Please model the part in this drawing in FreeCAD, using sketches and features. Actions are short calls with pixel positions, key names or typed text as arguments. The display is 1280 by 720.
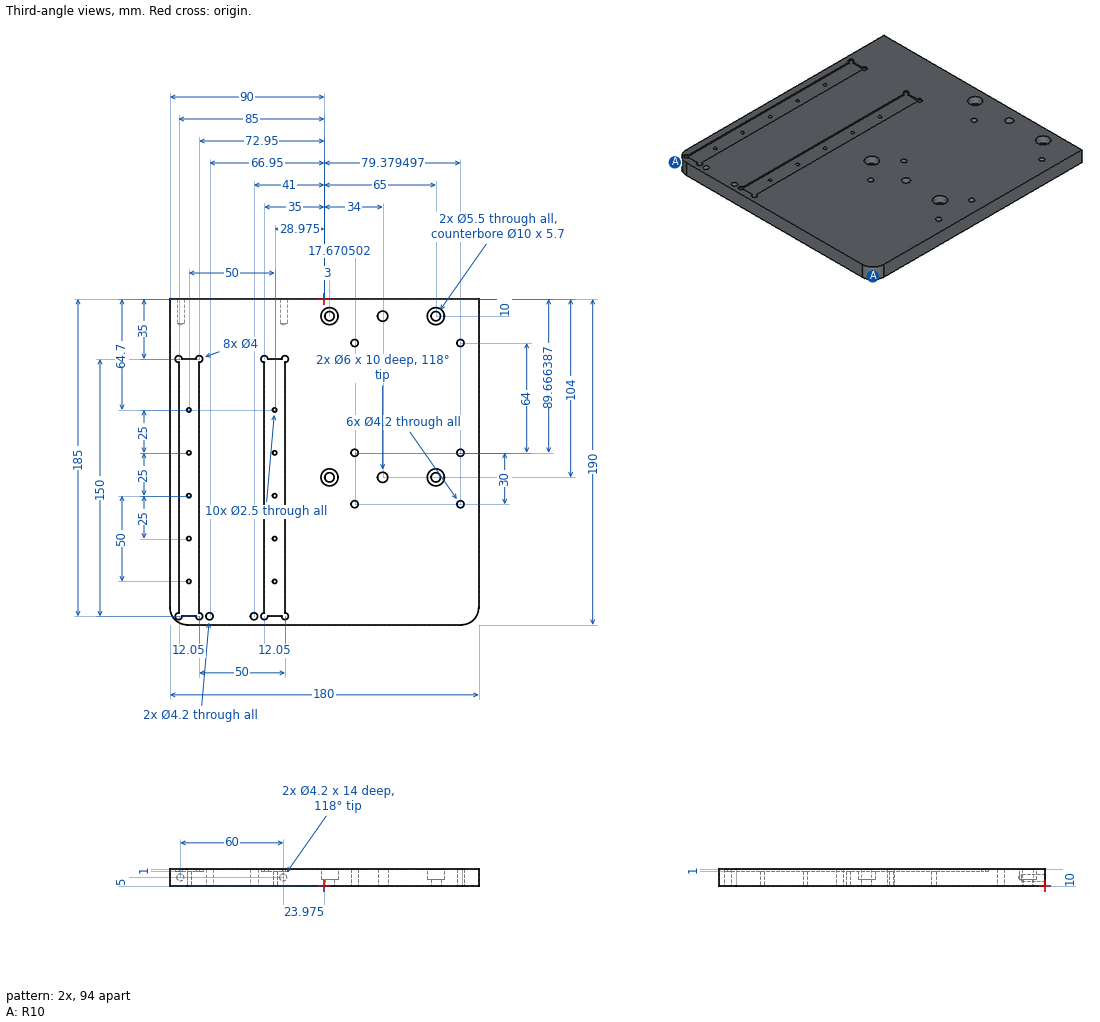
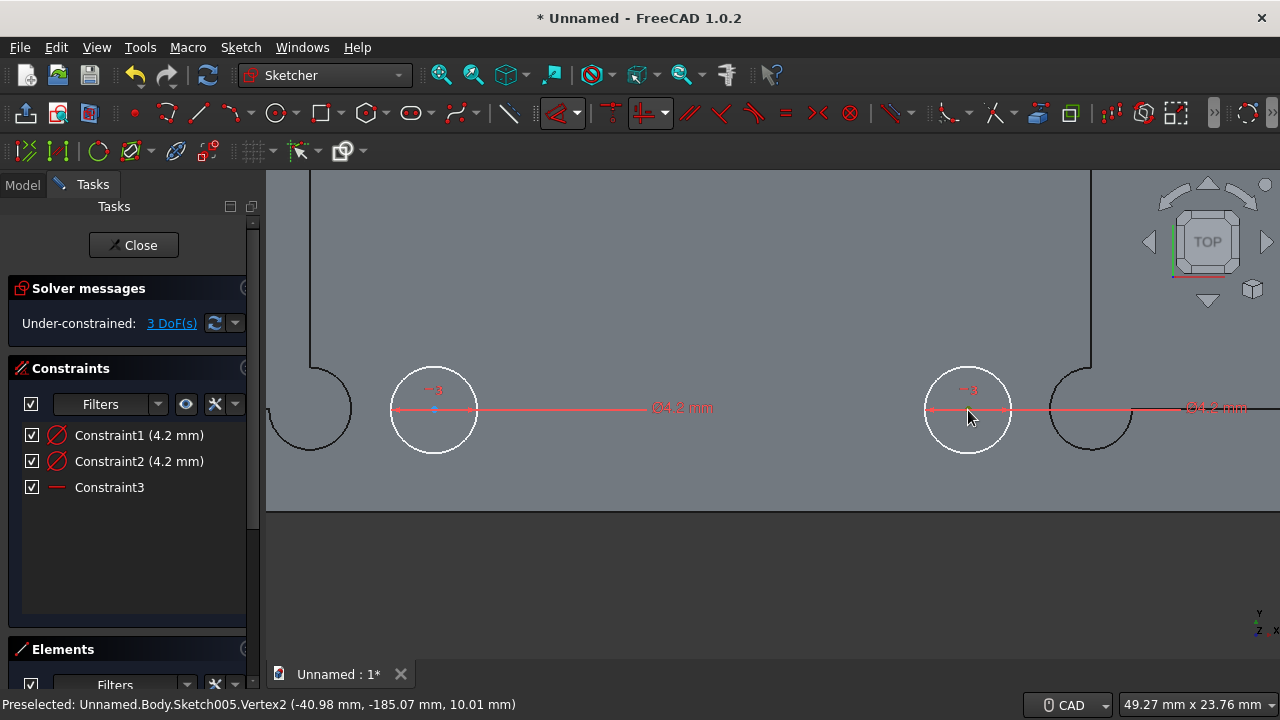
click(580, 114)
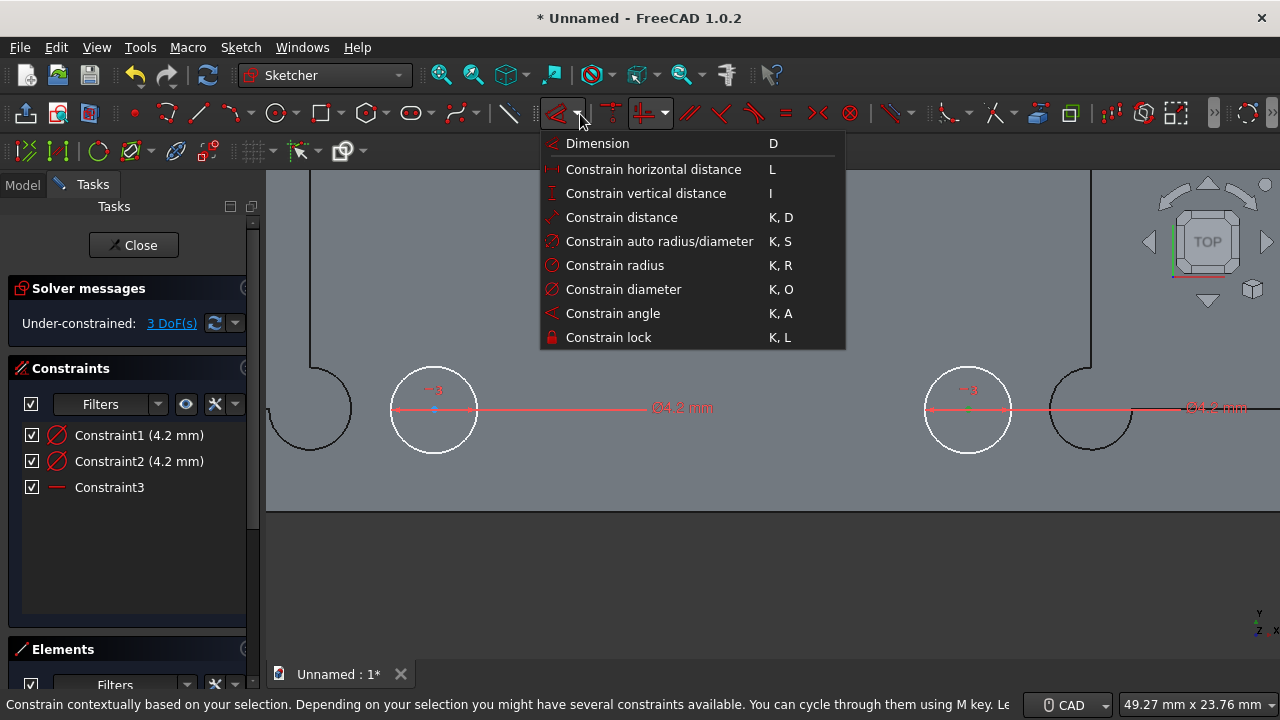
click(693, 169)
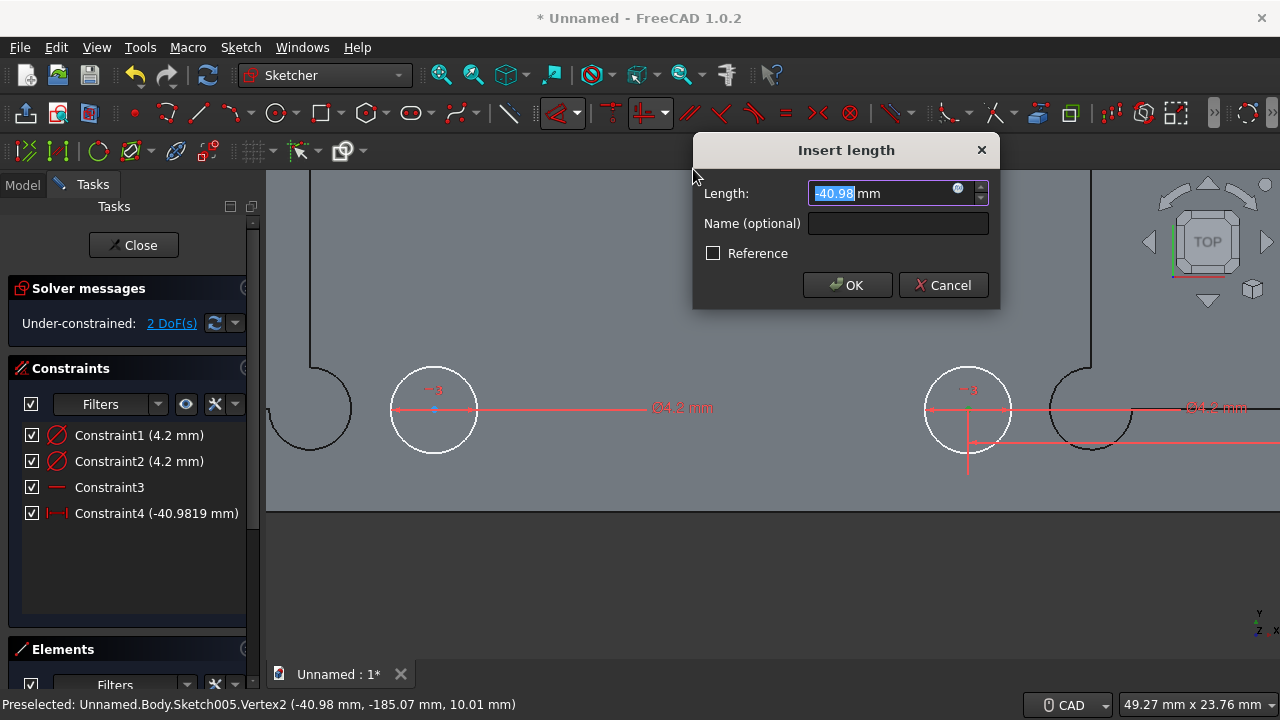
text(-41)
key(Return)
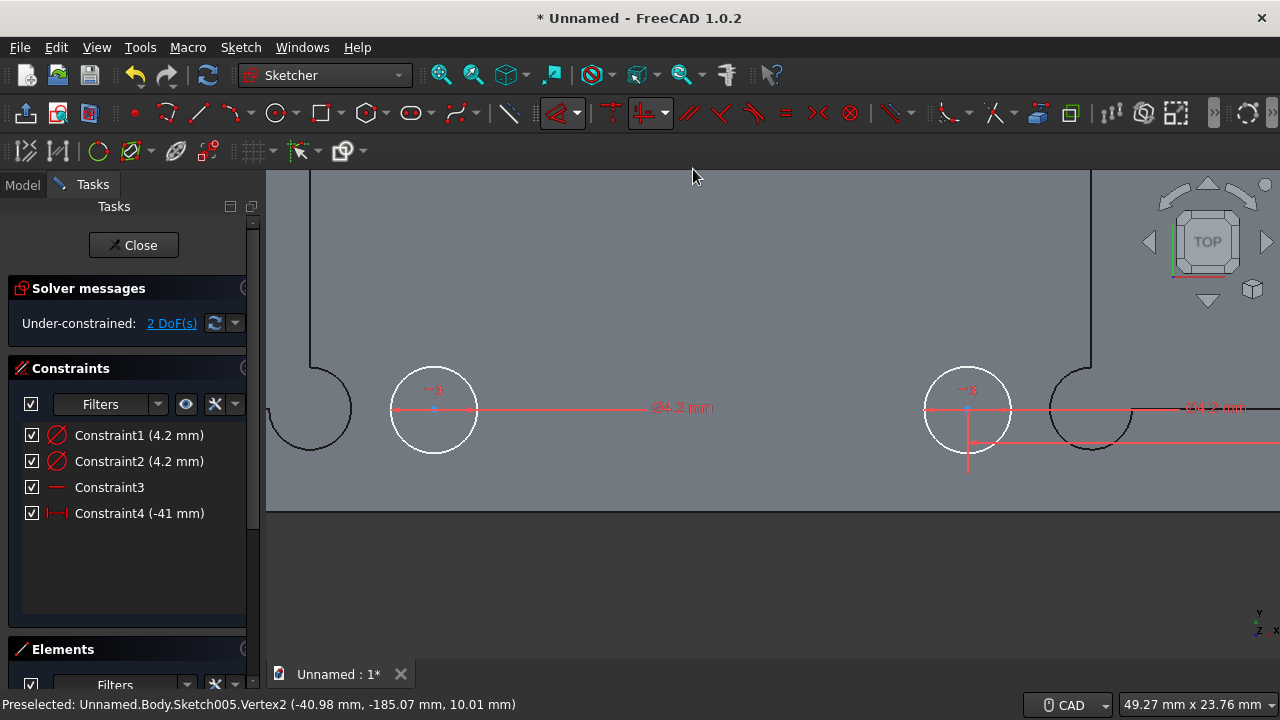
click(434, 410)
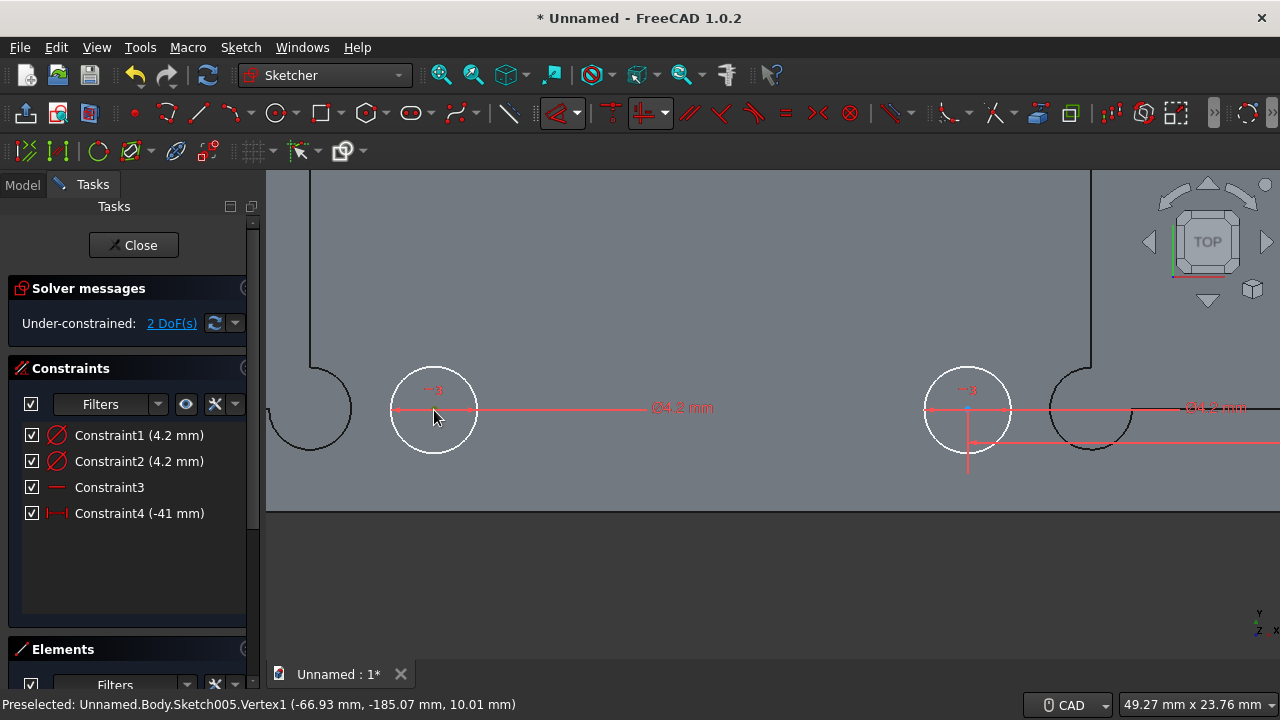
key(i)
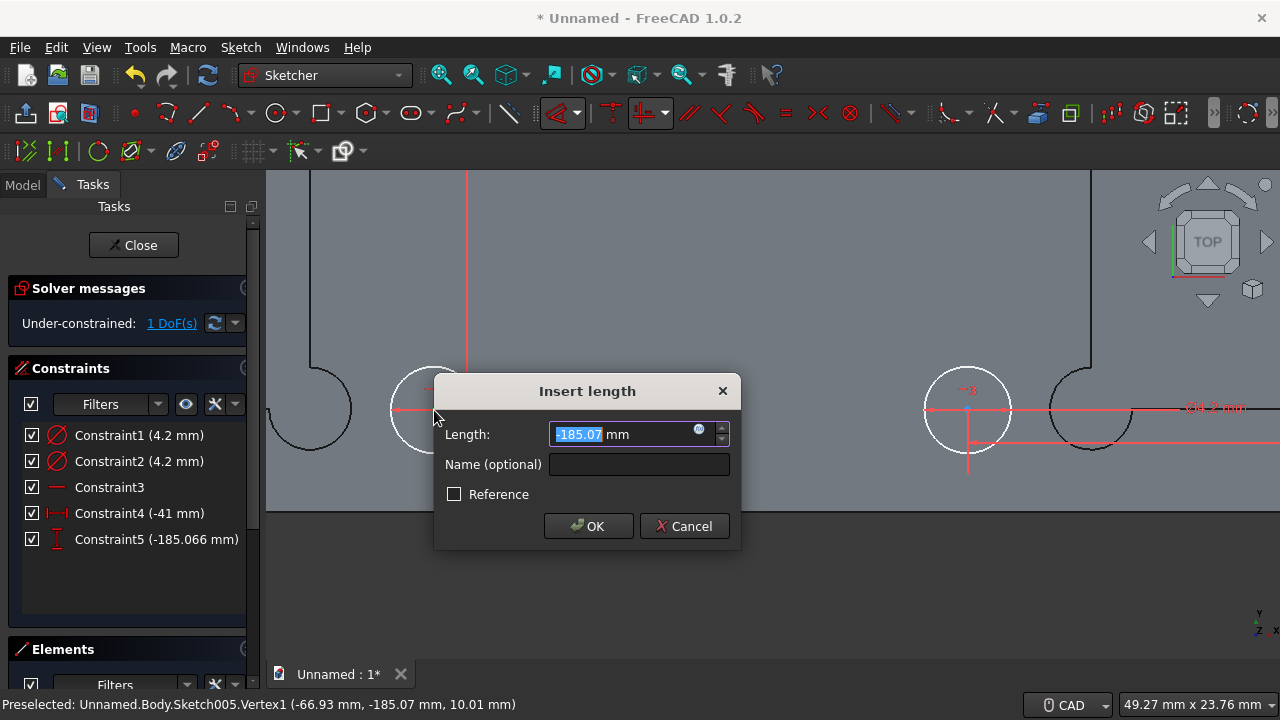
text(-185)
key(Return)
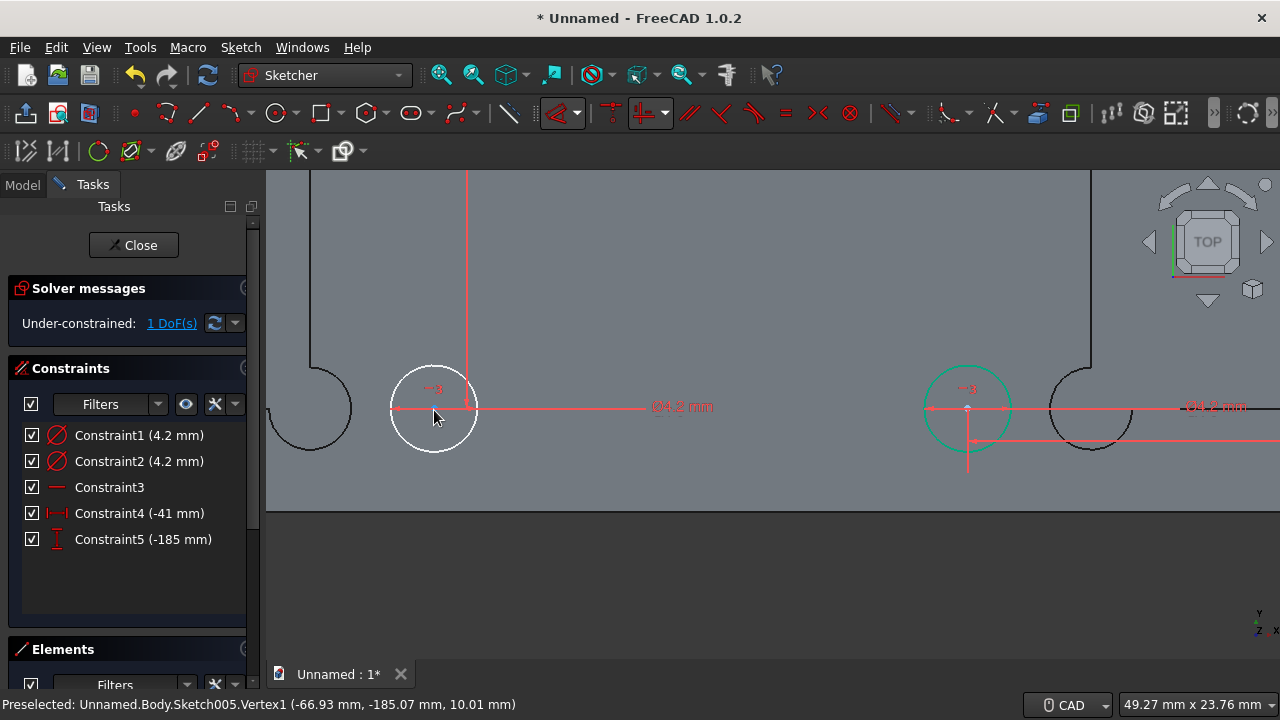
click(434, 409)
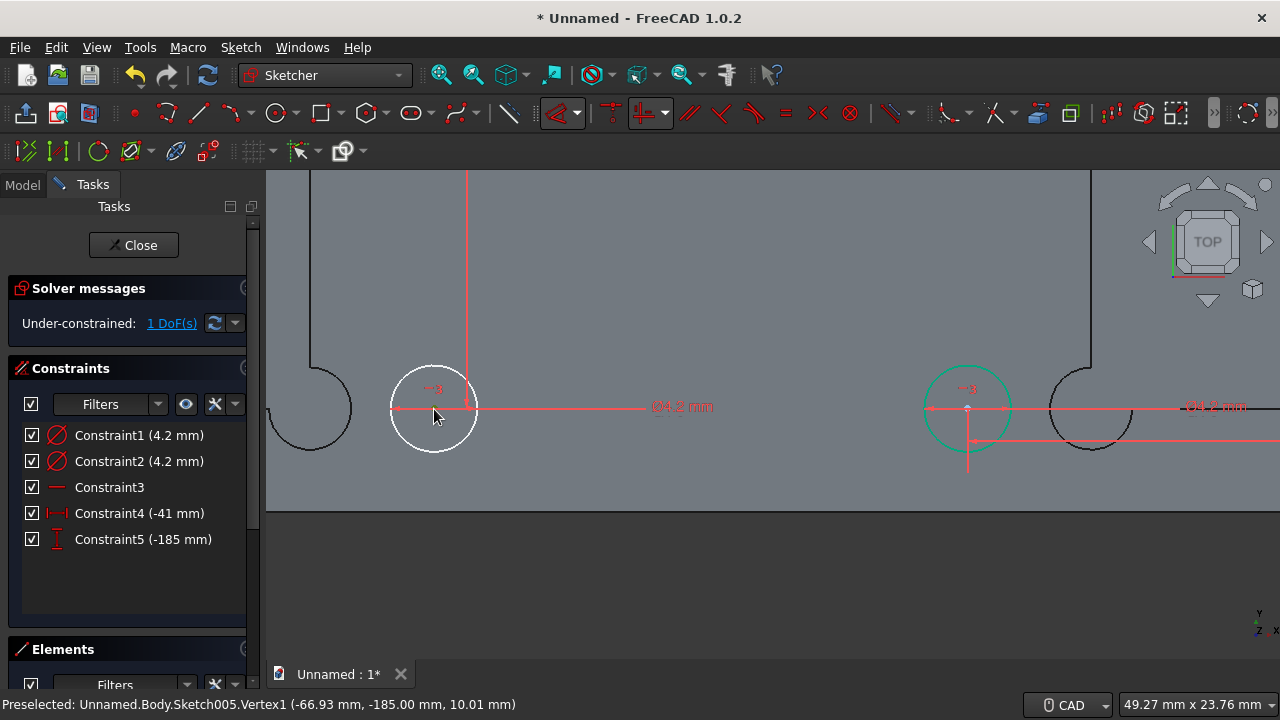
key(l)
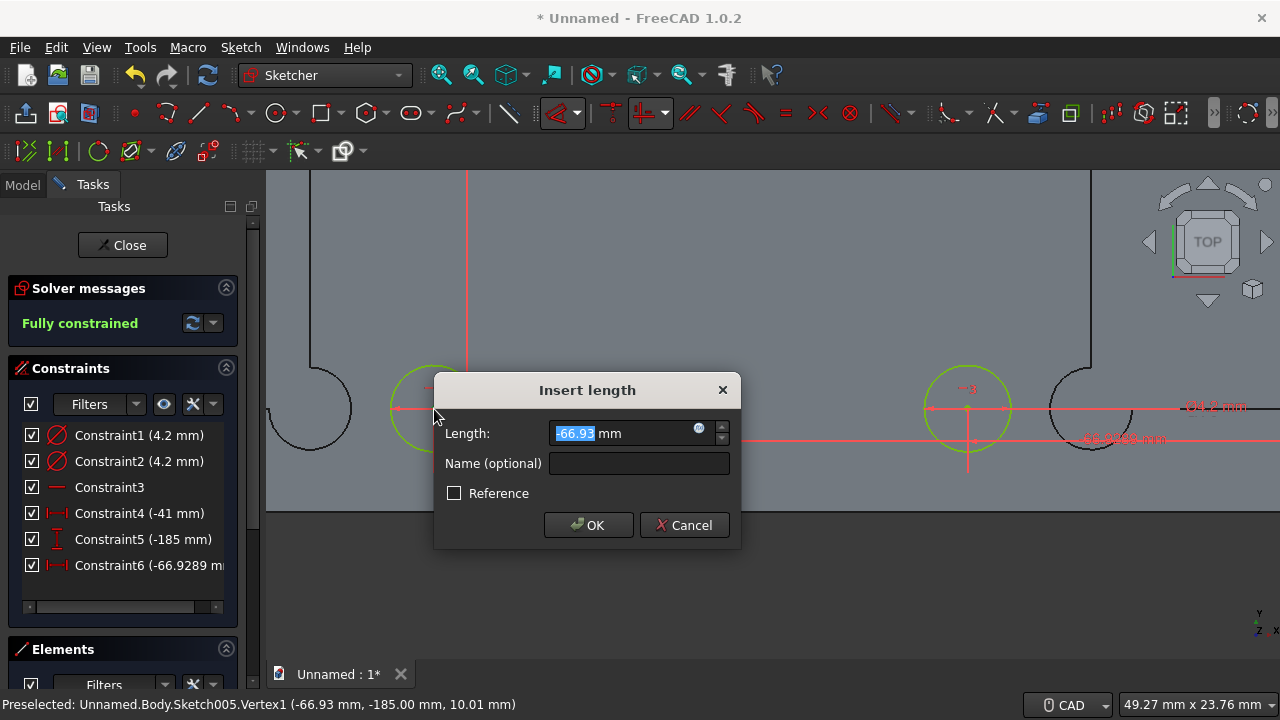
text(-66.95)
key(Return)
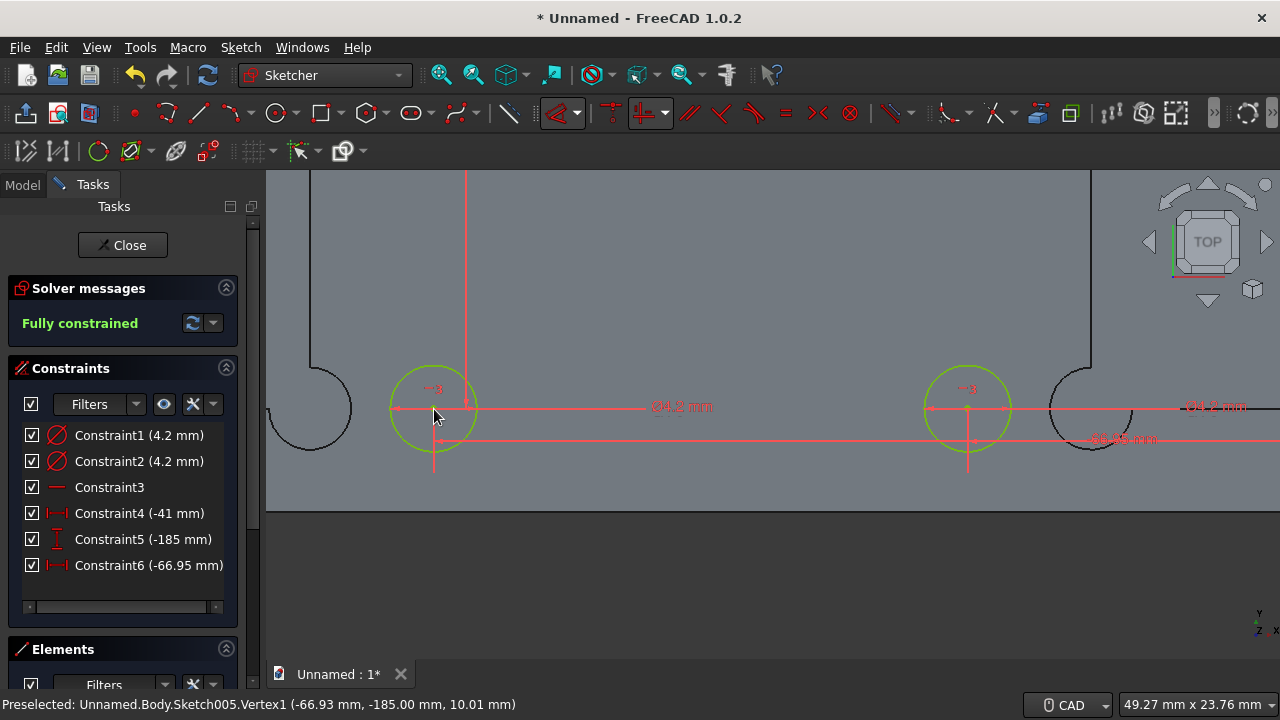
click(123, 245)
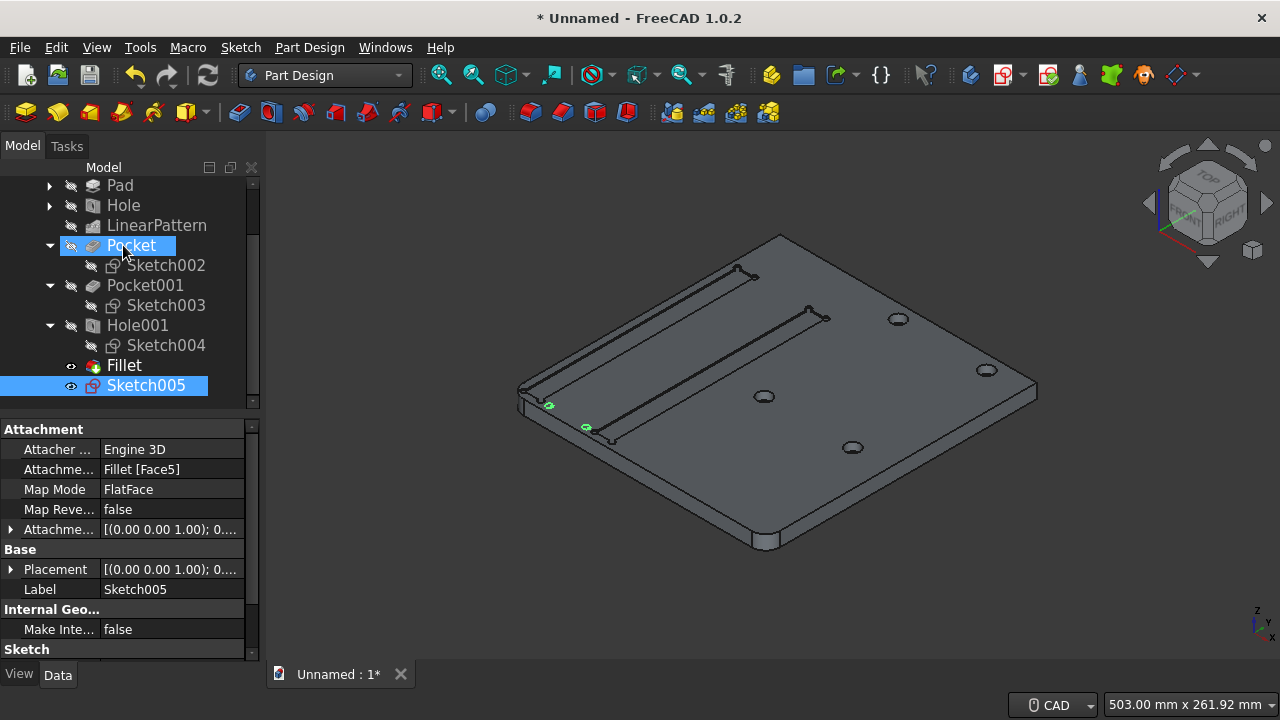
click(272, 112)